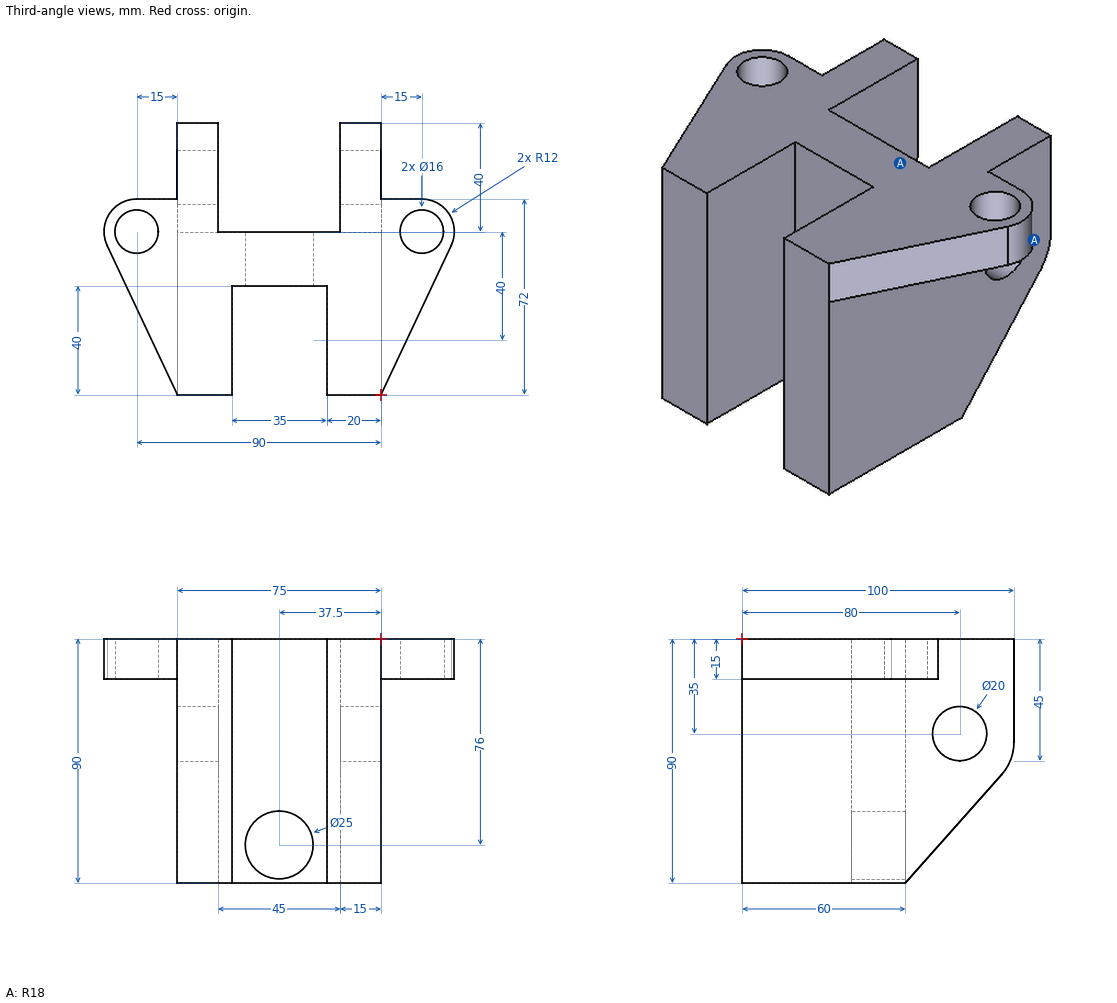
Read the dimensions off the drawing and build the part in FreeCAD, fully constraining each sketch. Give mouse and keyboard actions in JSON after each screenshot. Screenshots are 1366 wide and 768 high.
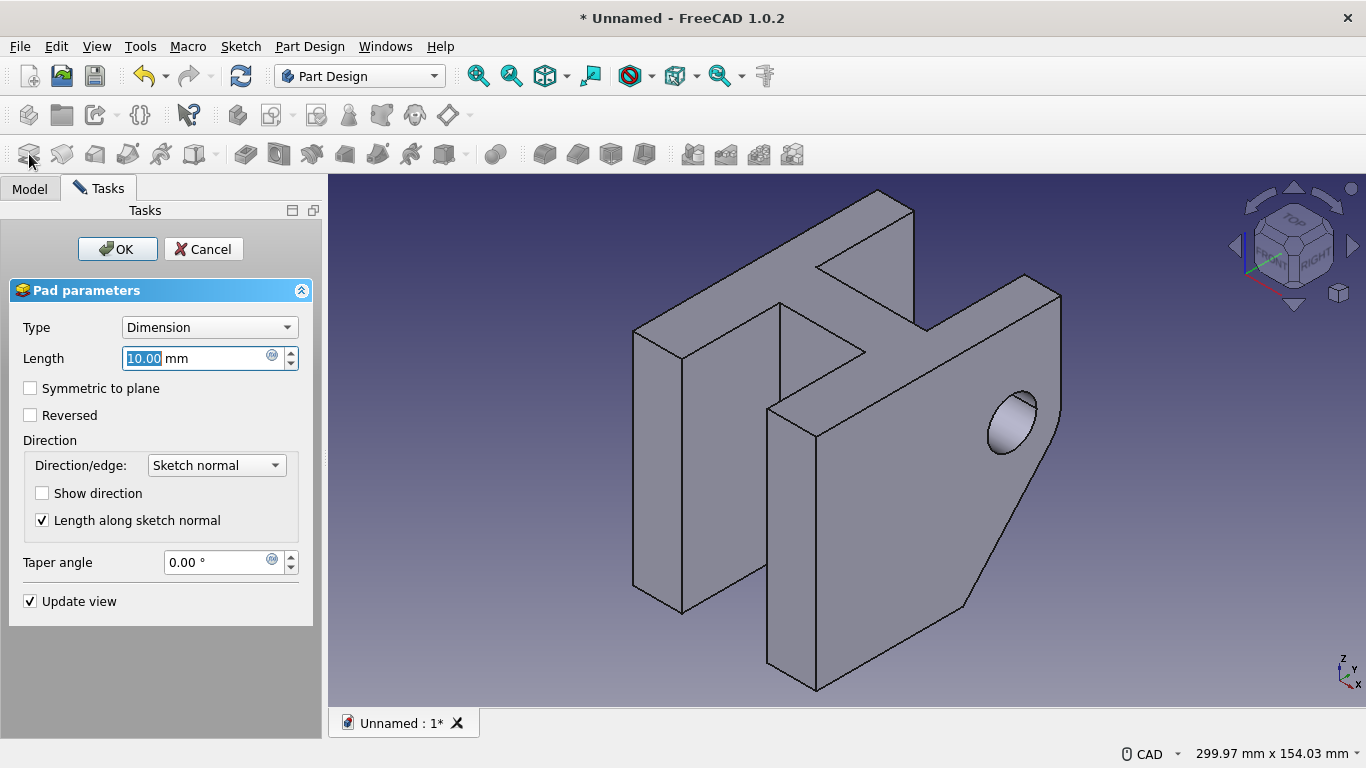
{"action": "type", "text": "15"}
{"action": "key", "text": "Tab"}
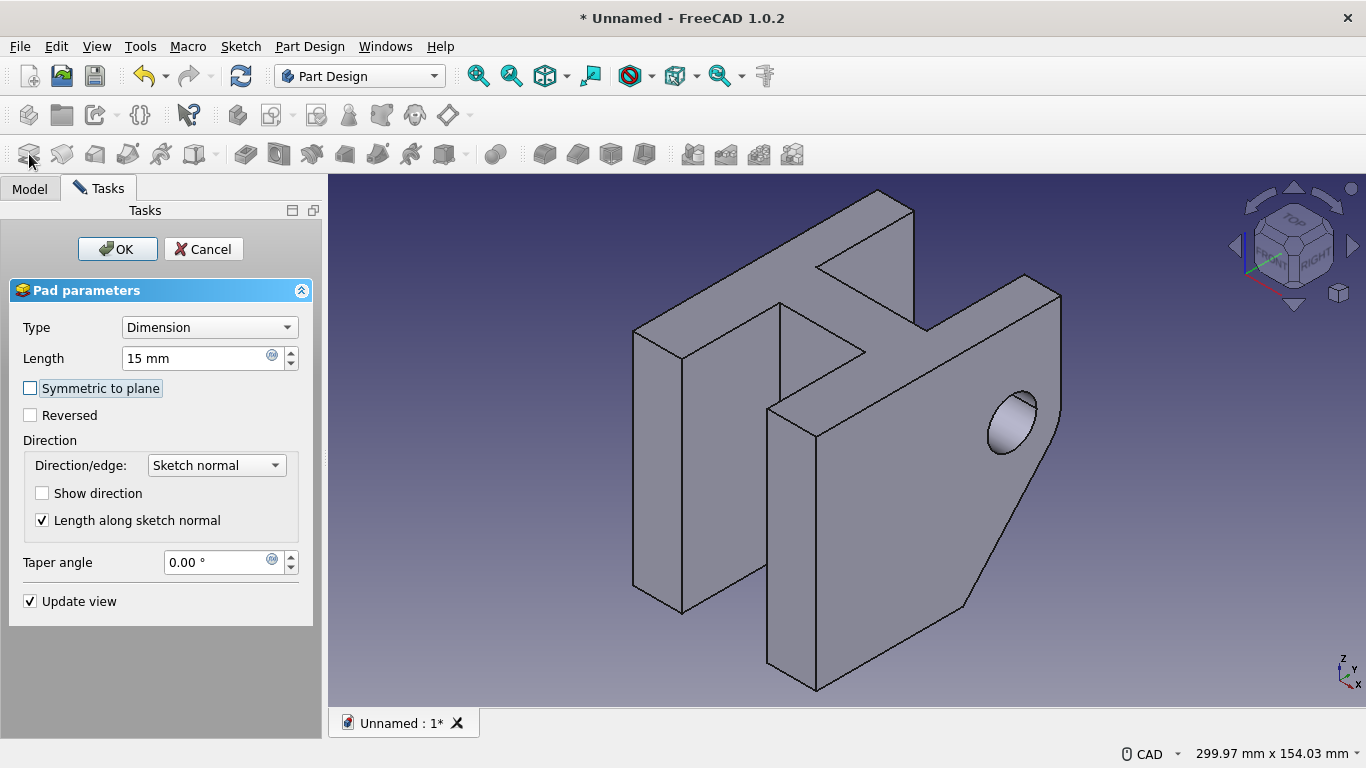
{"action": "left_click", "coordinate": [31, 415]}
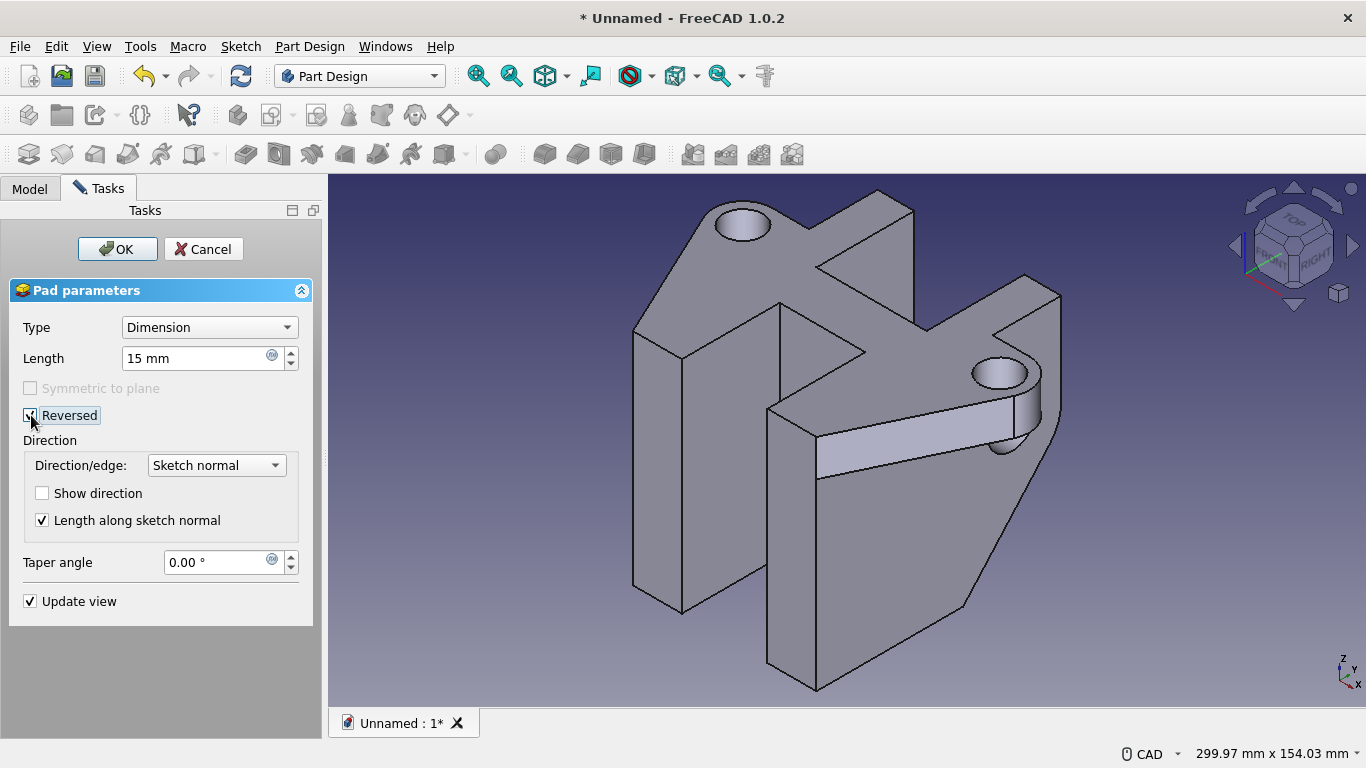
{"action": "left_click", "coordinate": [118, 249]}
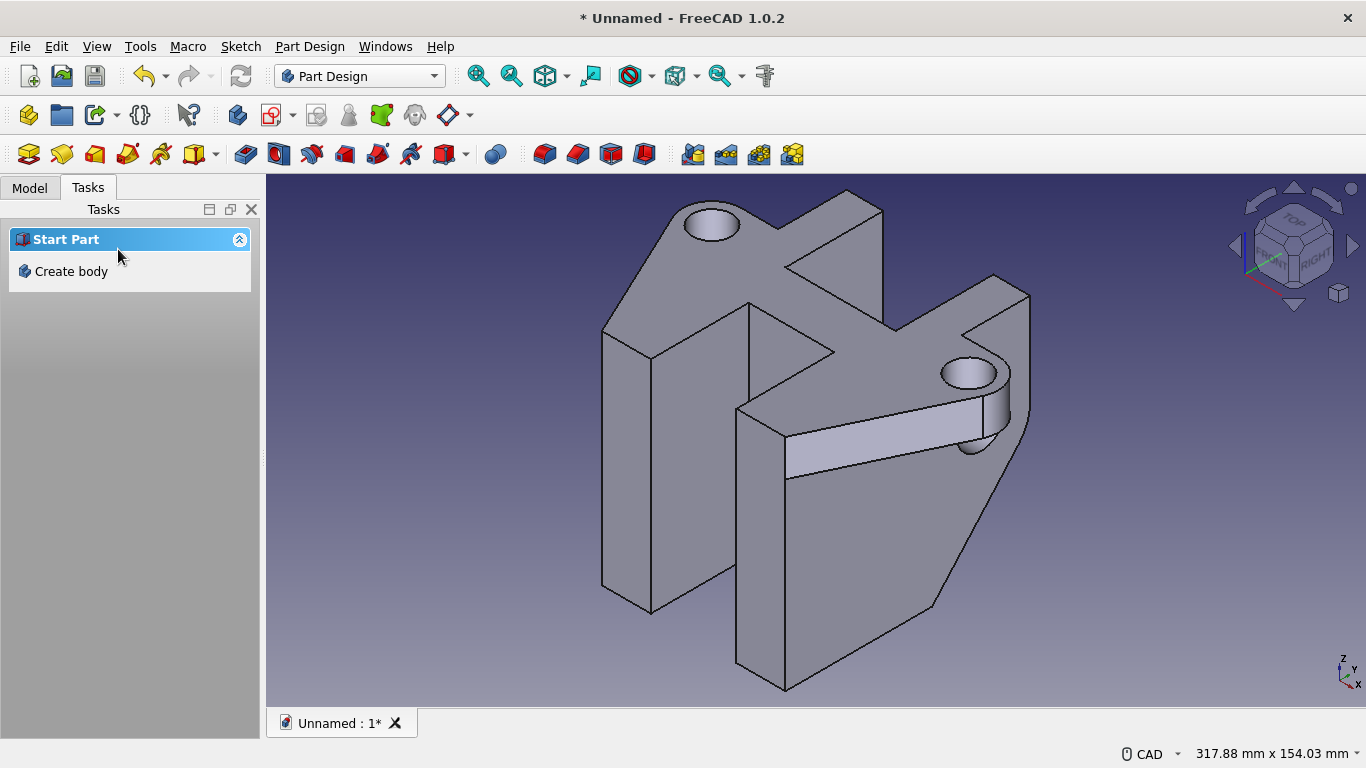
{"action": "left_click", "coordinate": [479, 76]}